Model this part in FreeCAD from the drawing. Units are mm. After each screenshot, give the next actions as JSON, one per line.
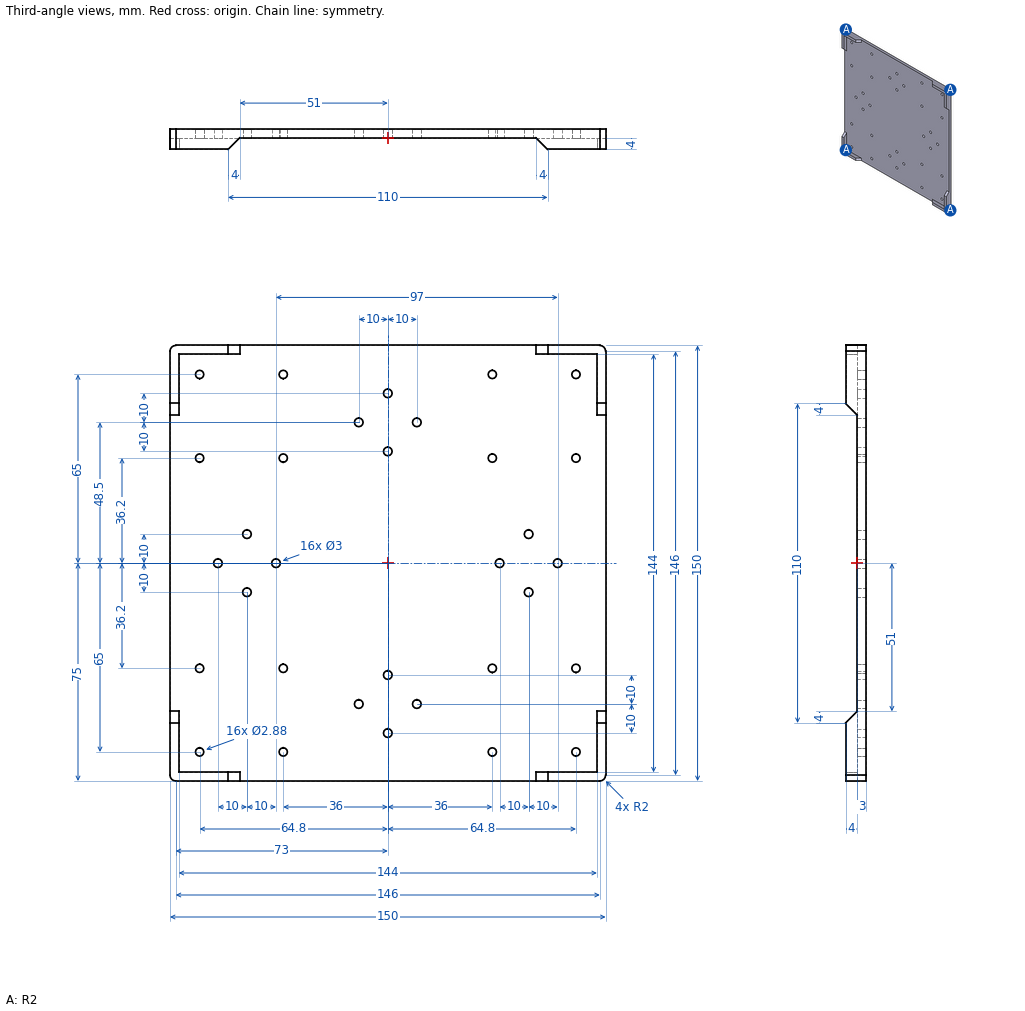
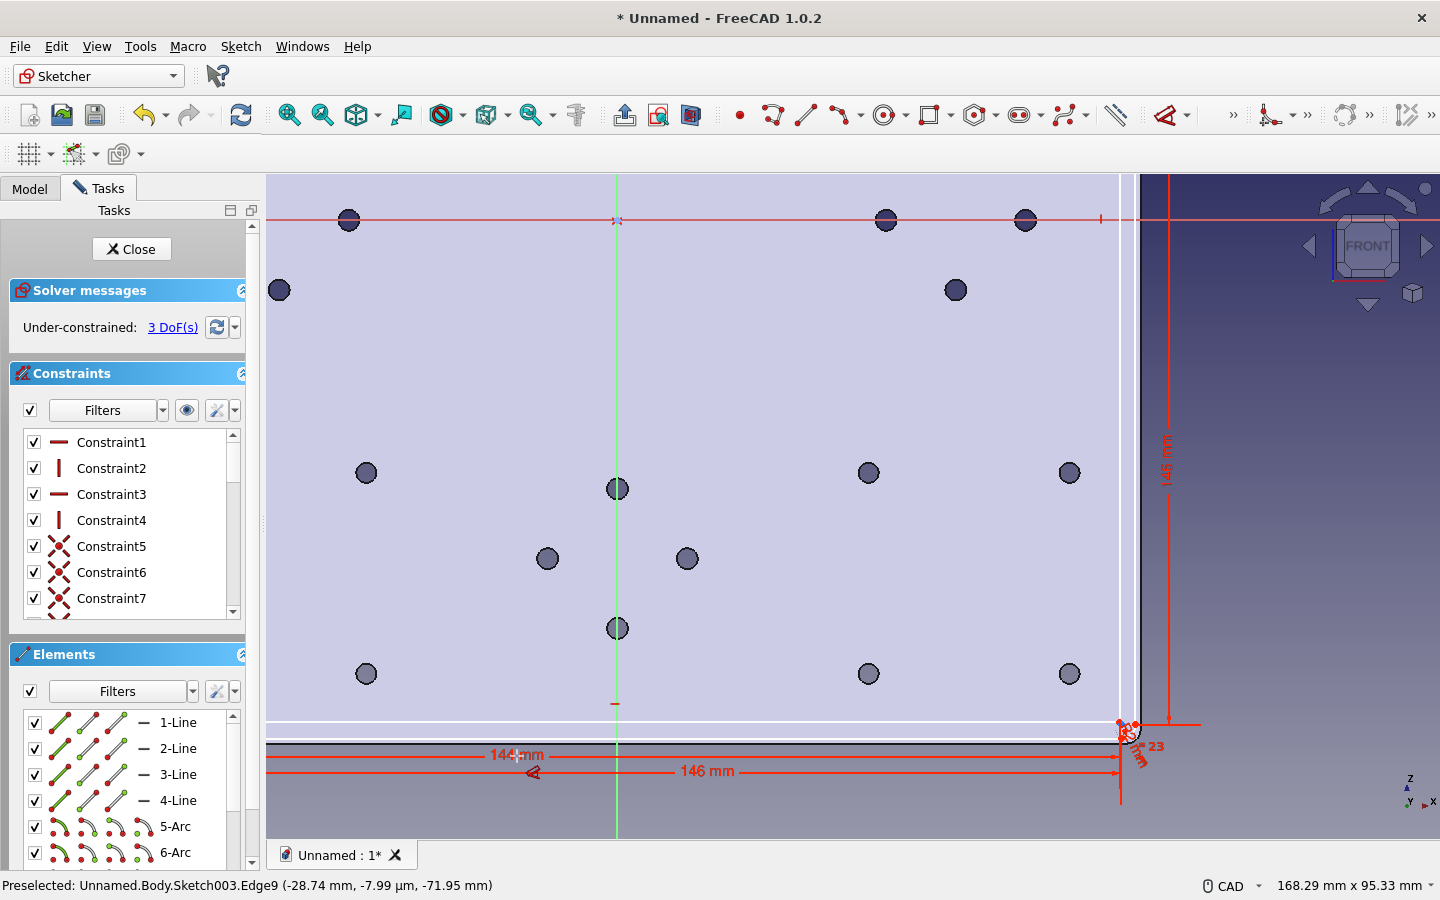
{"action": "left_click", "coordinate": [1120, 421]}
{"action": "left_click", "coordinate": [1154, 342]}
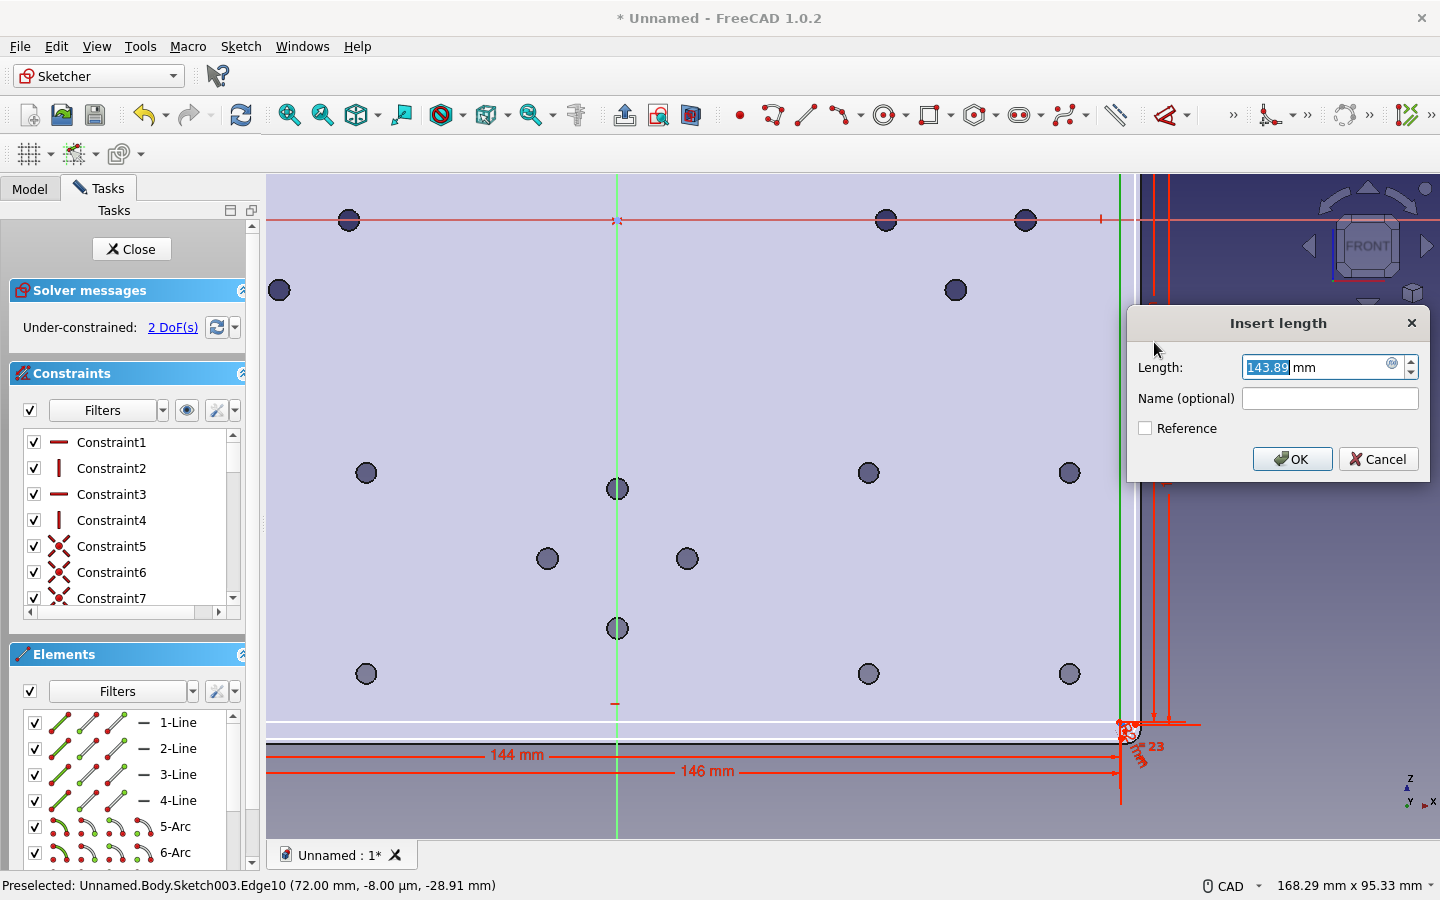
{"action": "type", "text": "144"}
{"action": "key", "text": "Return"}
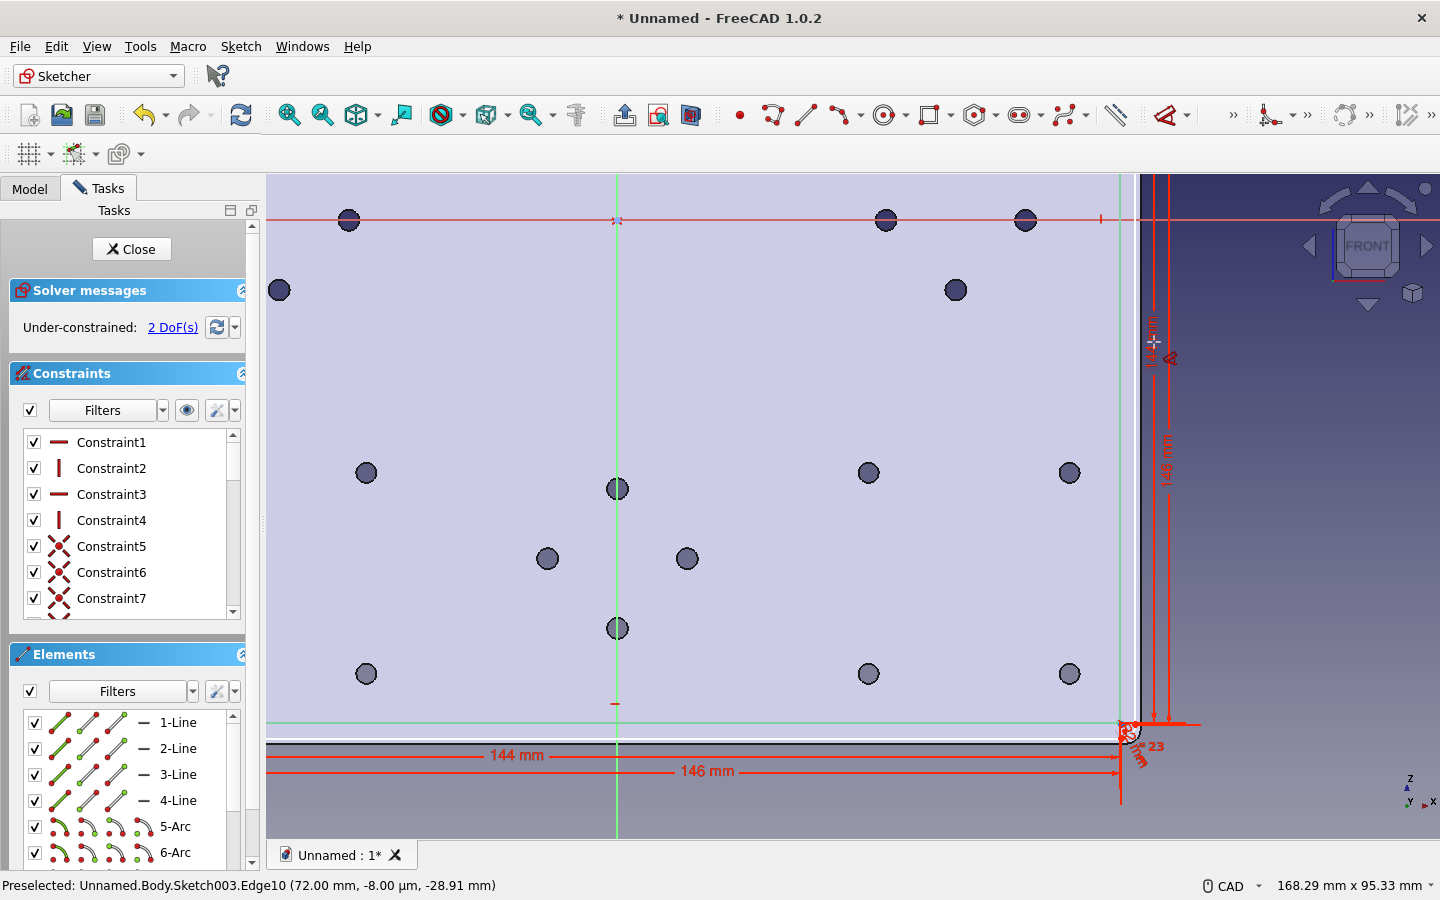
{"action": "scroll", "coordinate": [921, 740], "scroll_direction": "down", "scroll_amount": 4}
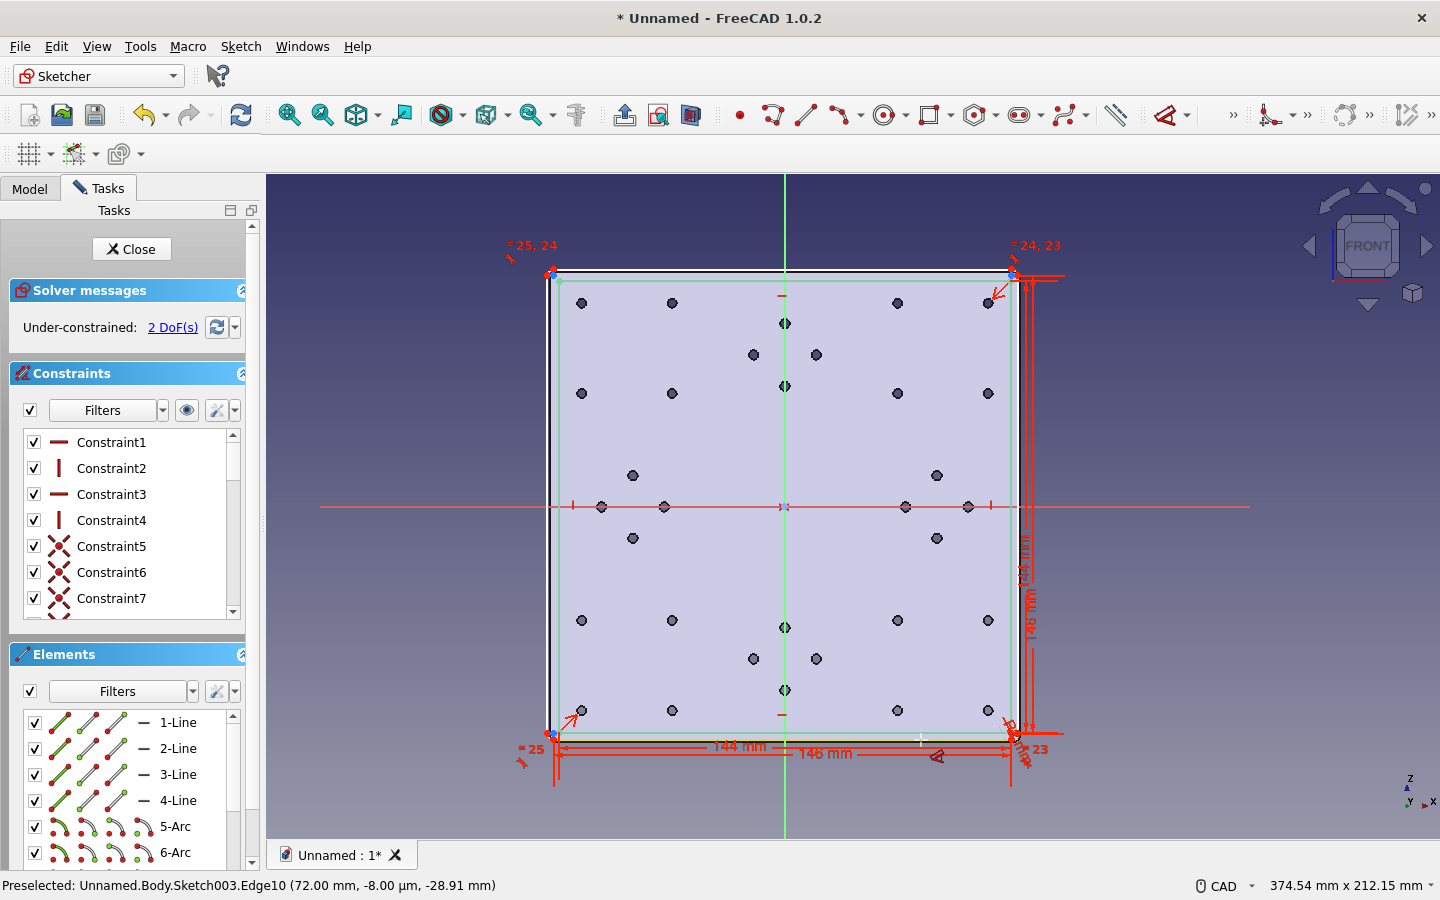
{"action": "scroll", "coordinate": [554, 740], "scroll_direction": "up", "scroll_amount": 4}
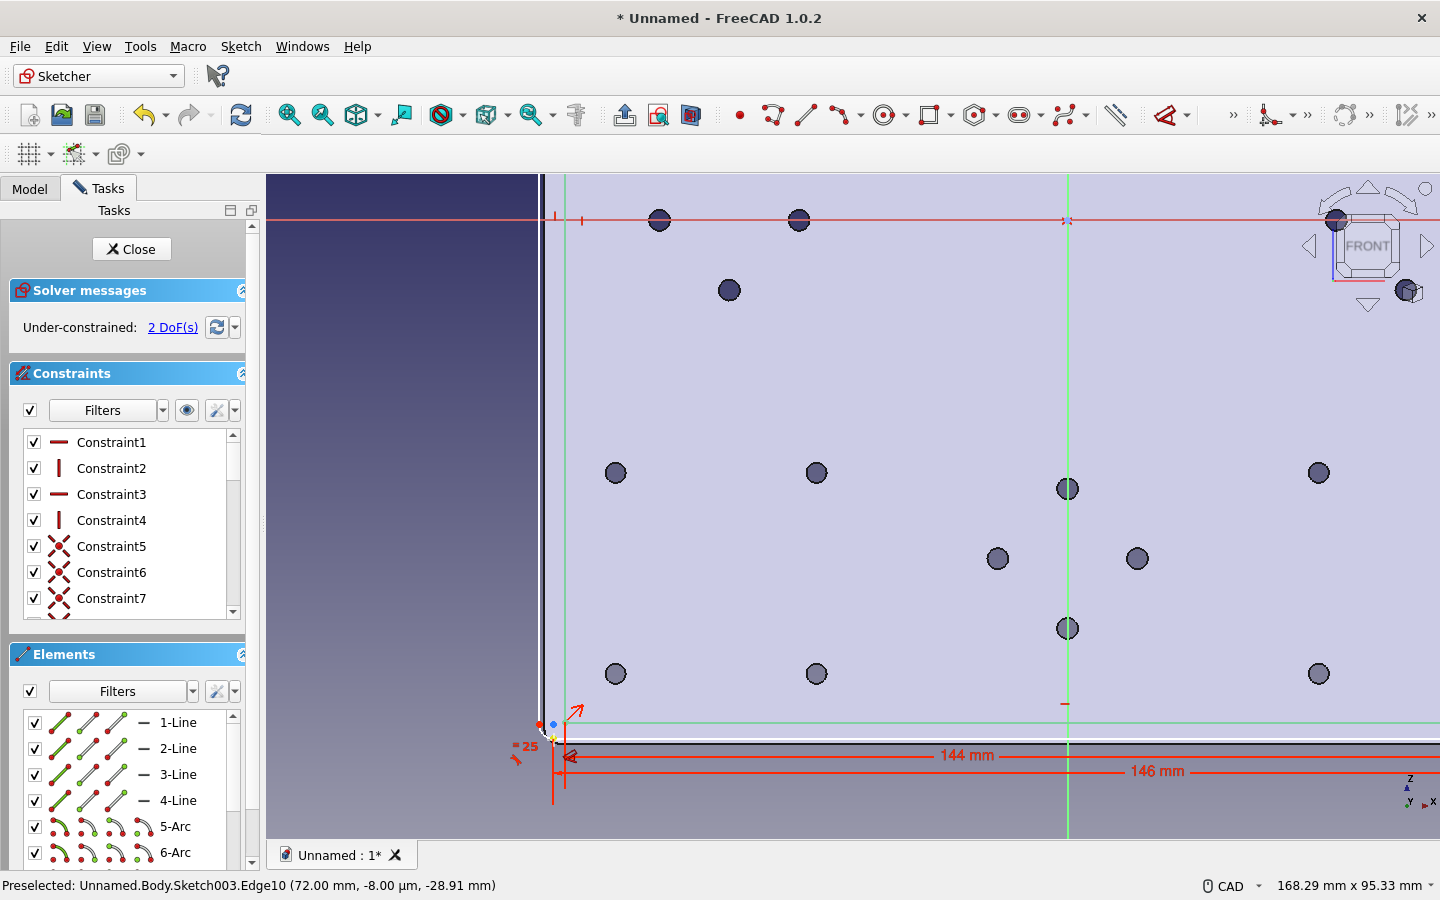
{"action": "left_click", "coordinate": [553, 739]}
{"action": "left_click", "coordinate": [810, 773]}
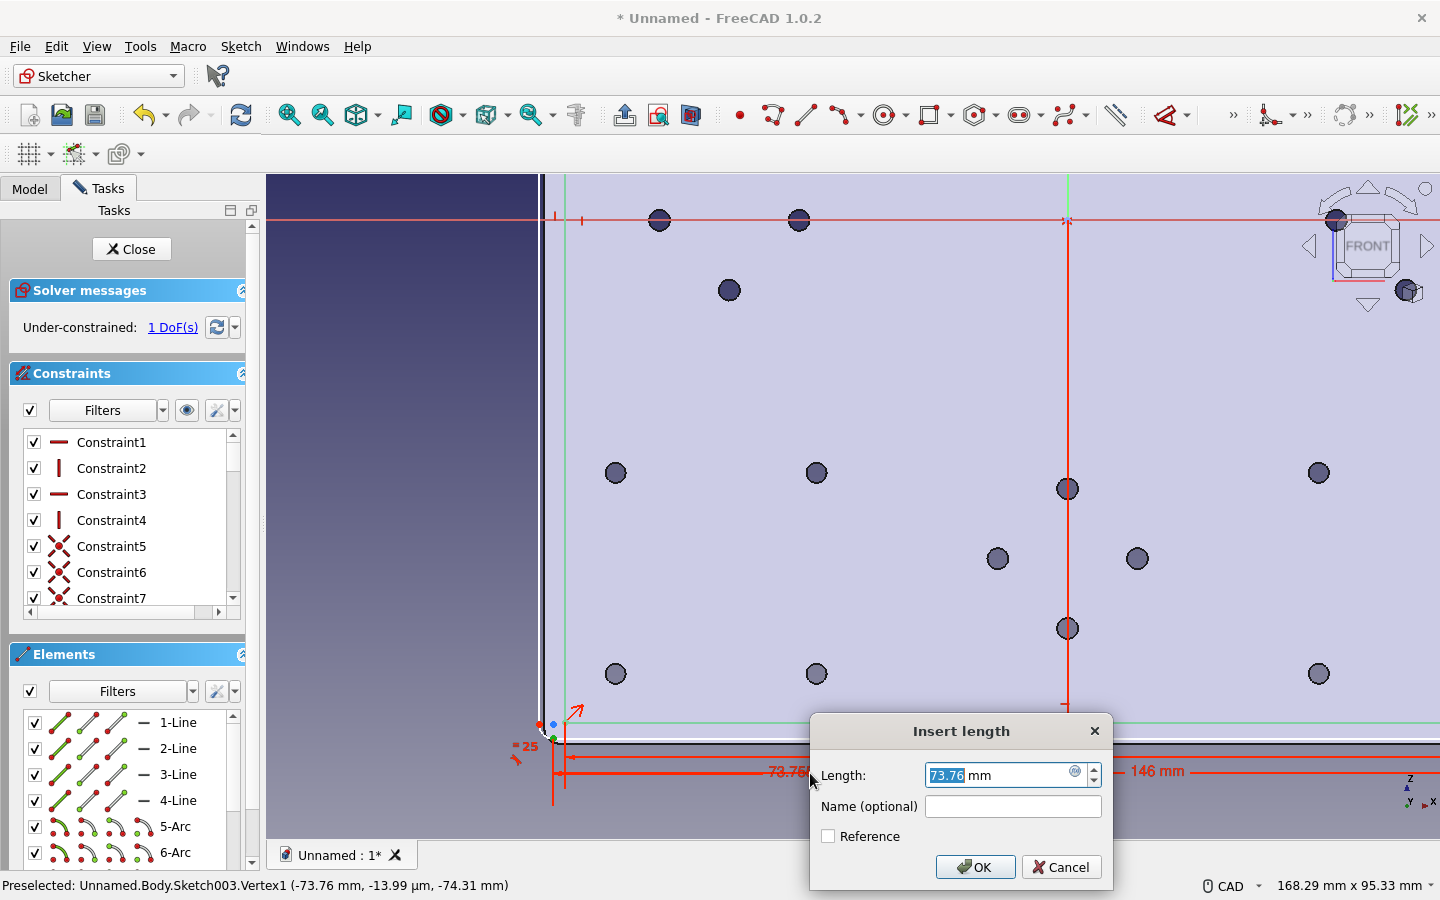
{"action": "type", "text": "73"}
{"action": "key", "text": "Return"}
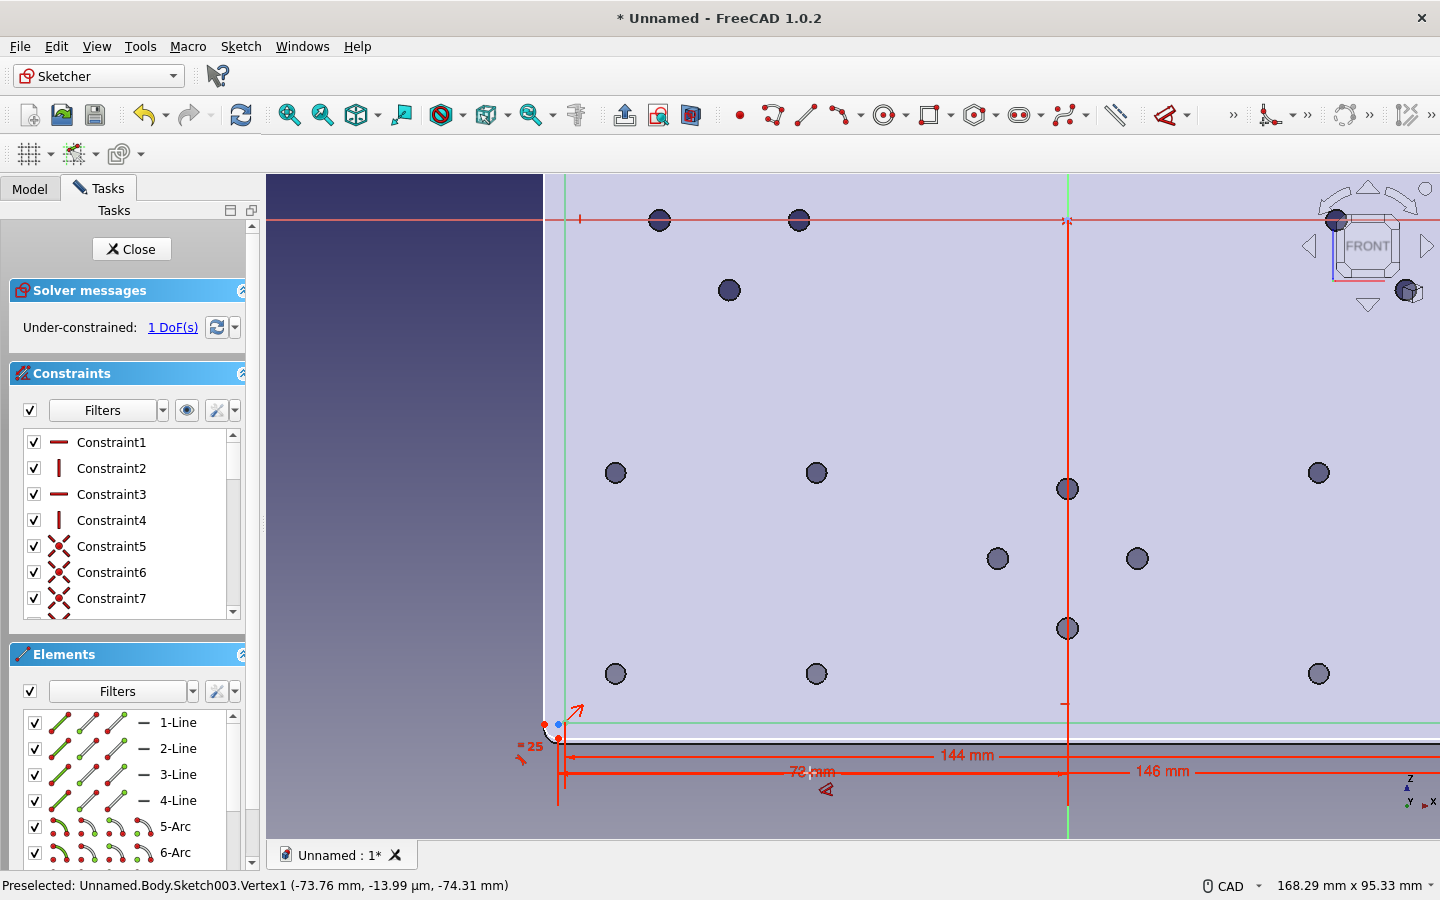
{"action": "left_click", "coordinate": [558, 739]}
{"action": "left_click", "coordinate": [524, 480]}